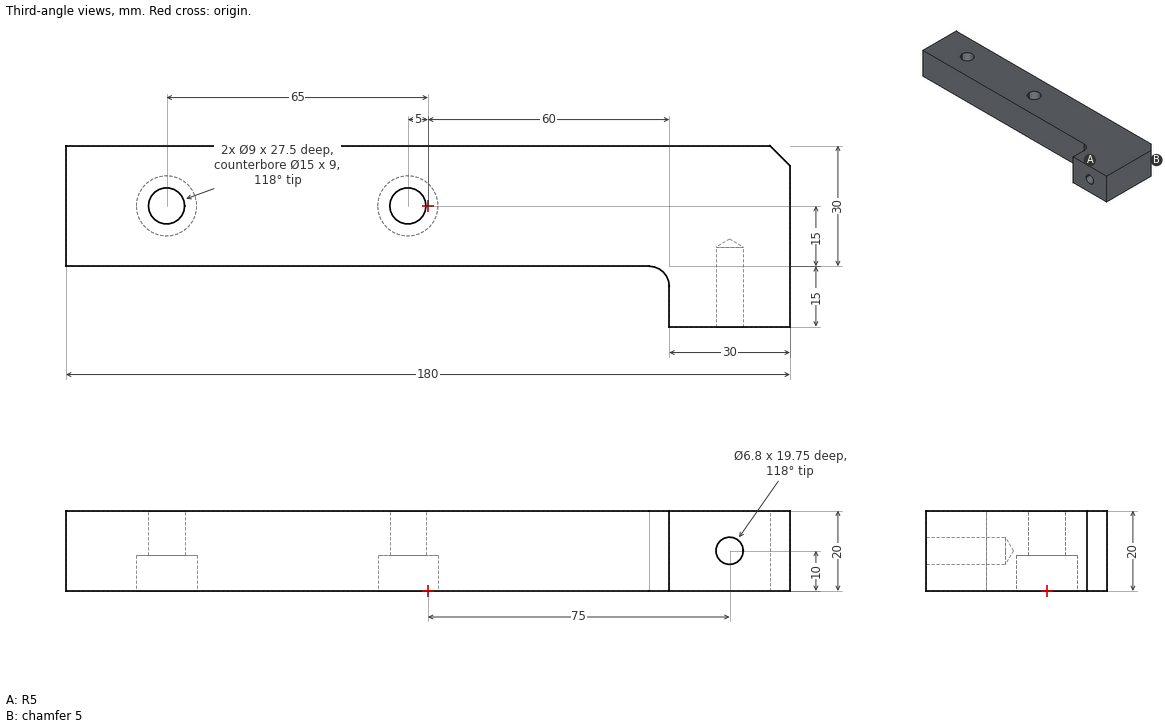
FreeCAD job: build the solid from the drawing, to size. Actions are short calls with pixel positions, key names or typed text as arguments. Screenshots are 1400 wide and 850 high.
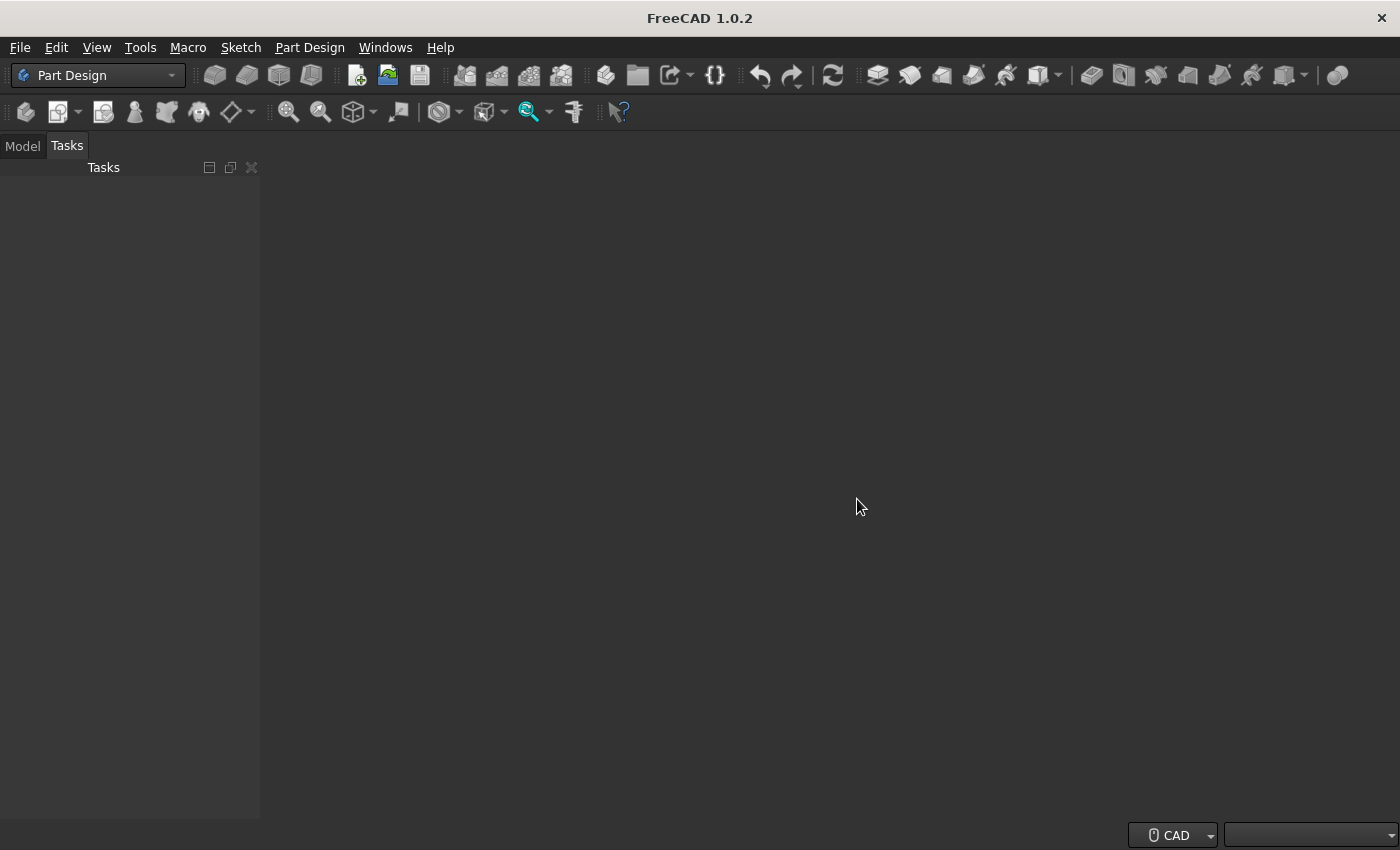
click(356, 76)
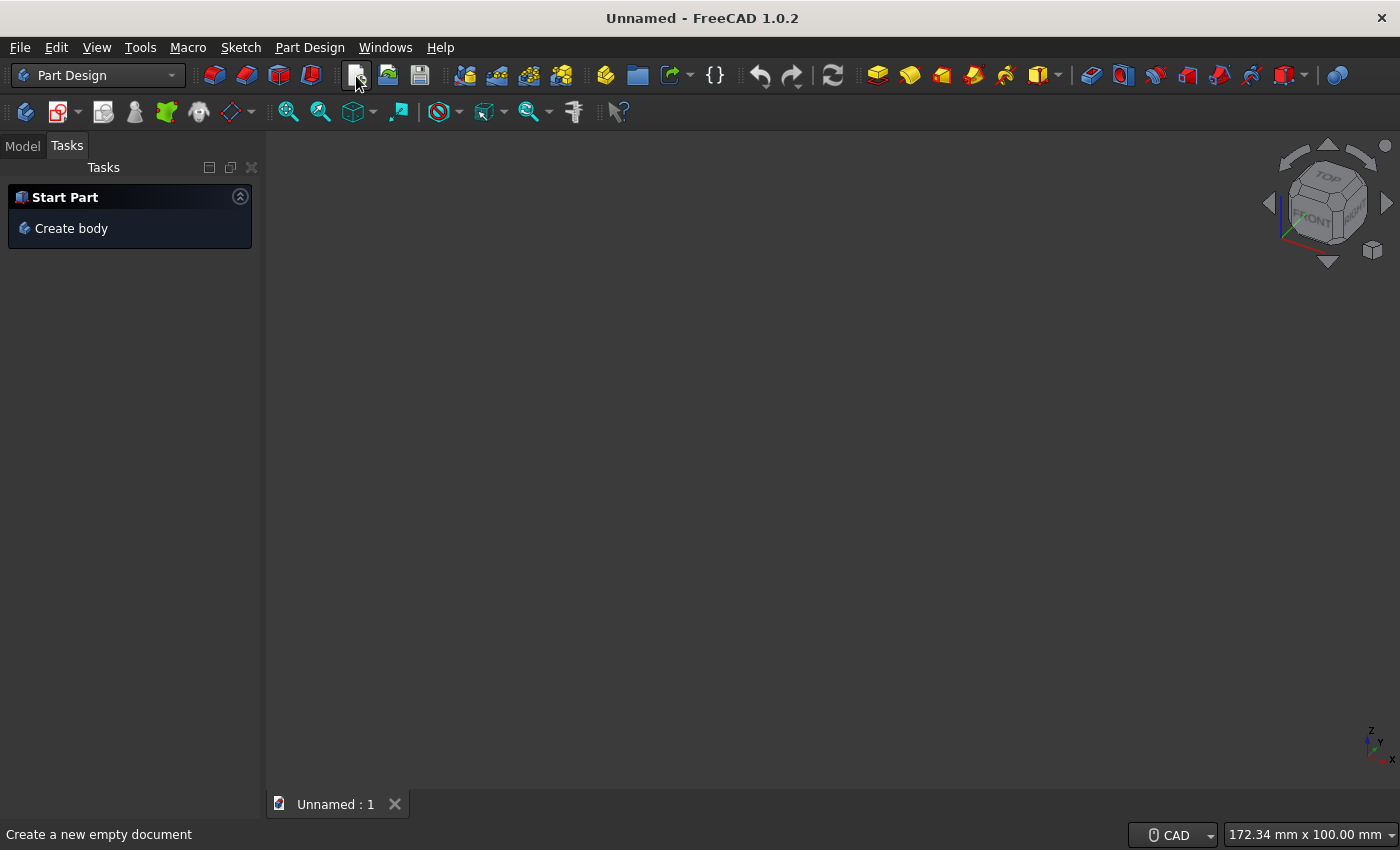
click(58, 112)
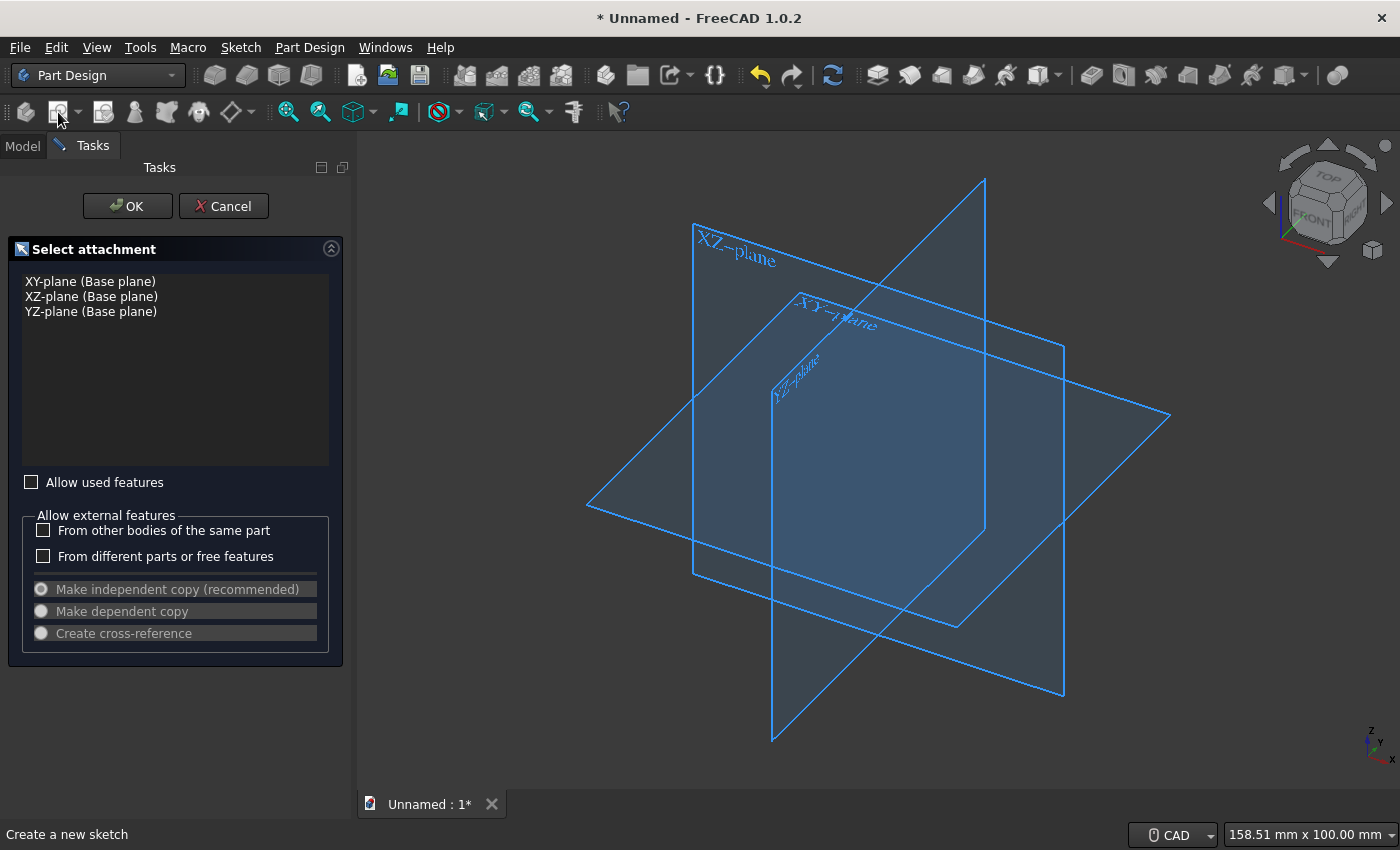
click(82, 282)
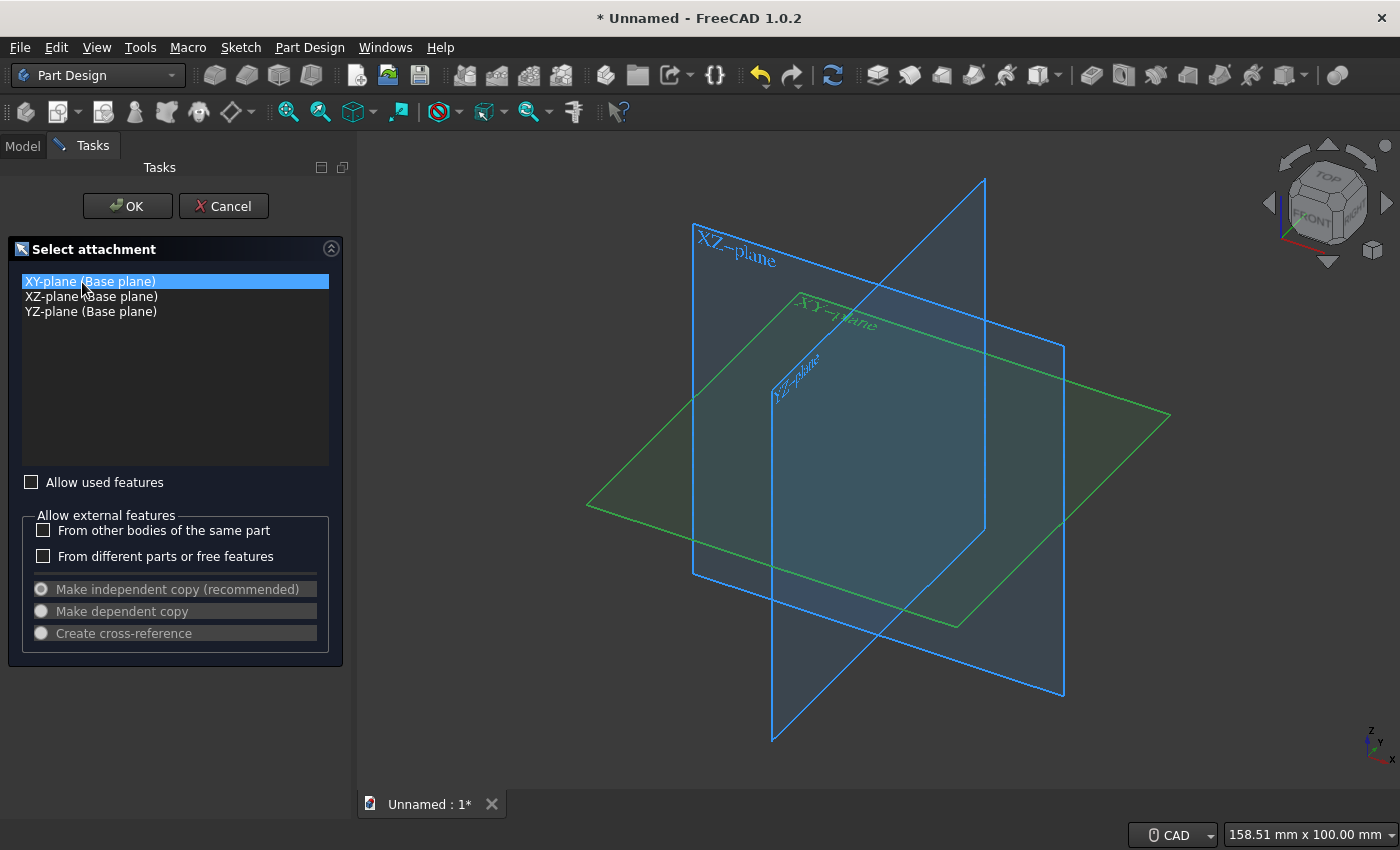
click(128, 206)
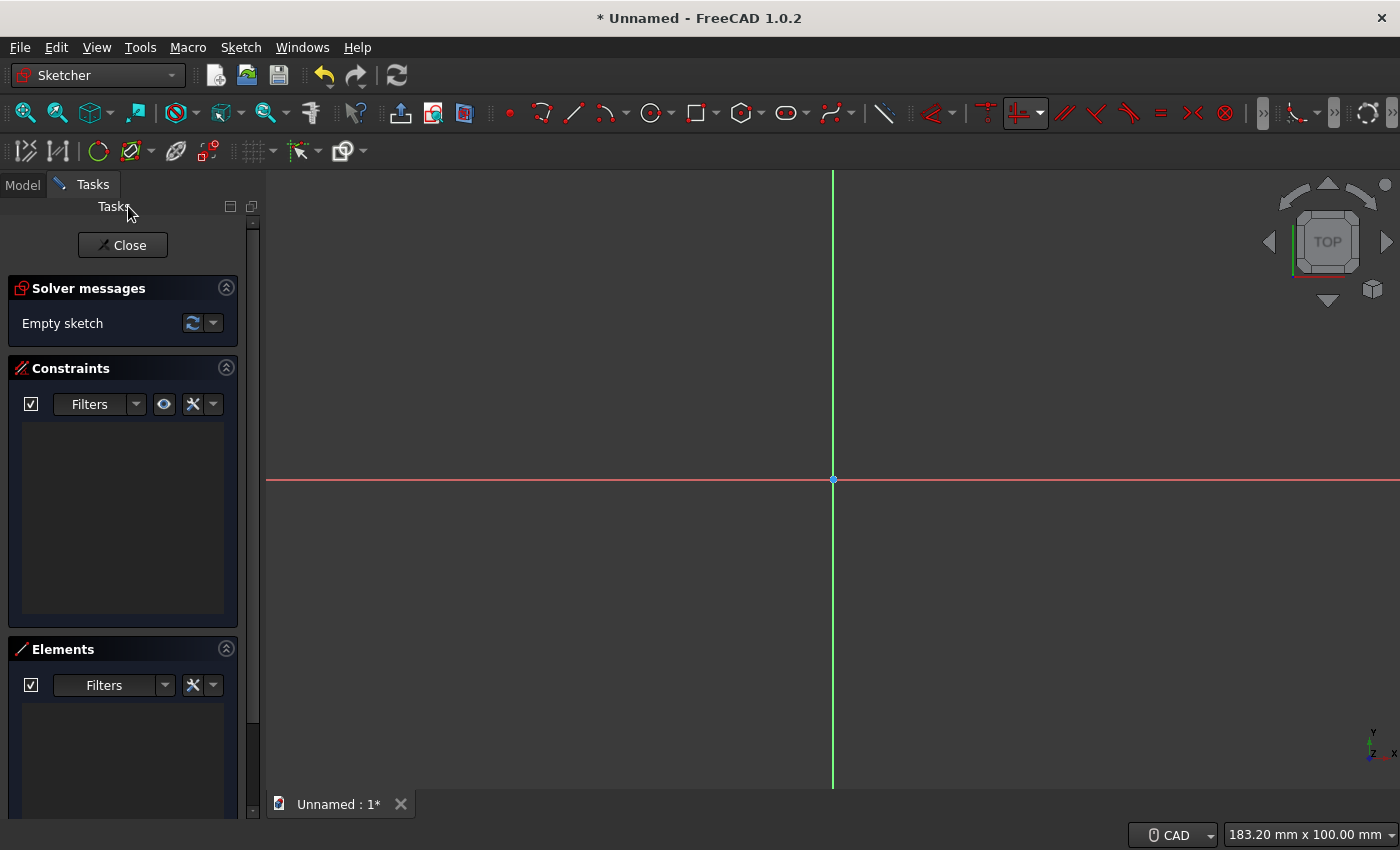
scroll(681, 479, down, 3)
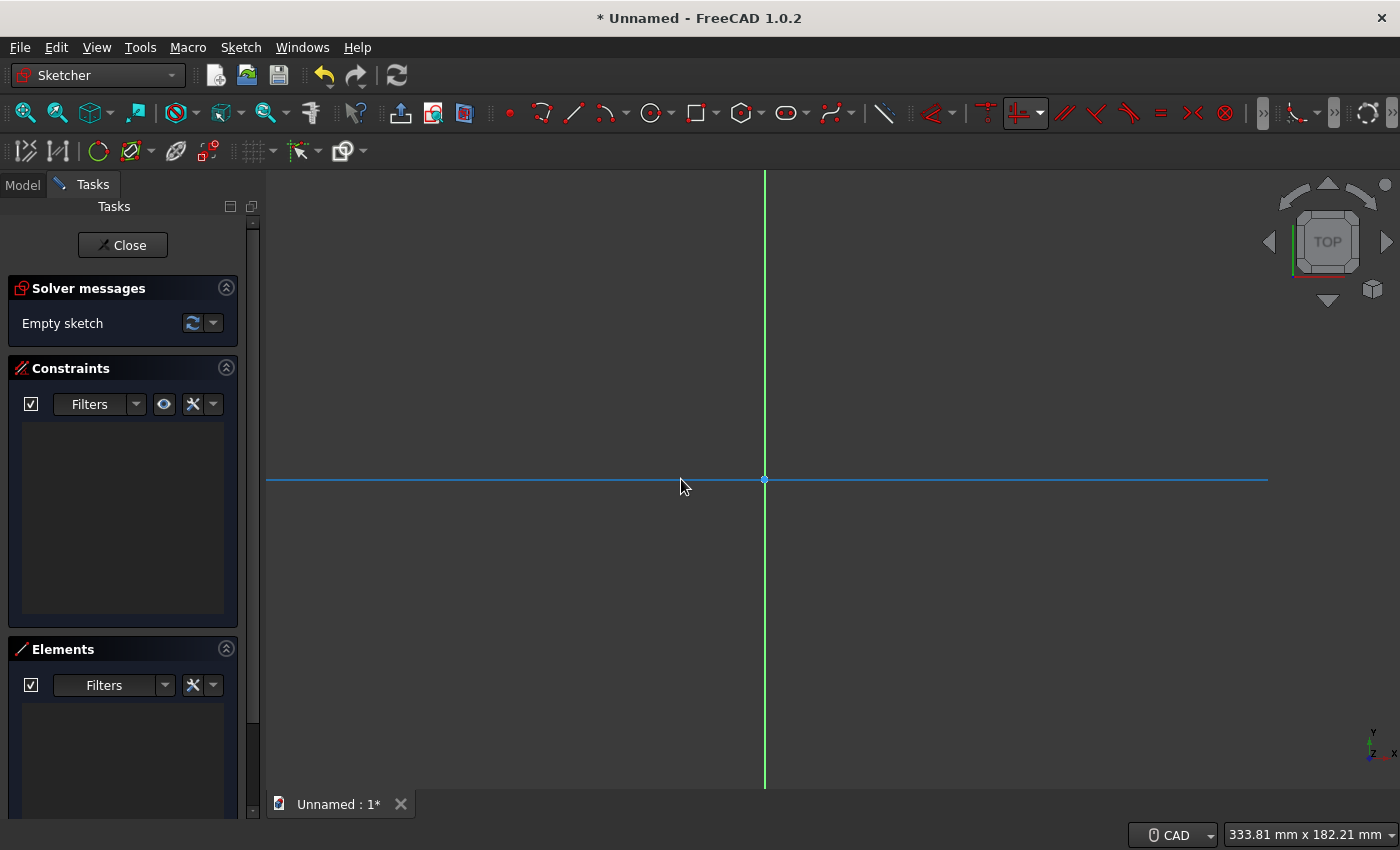
click(718, 114)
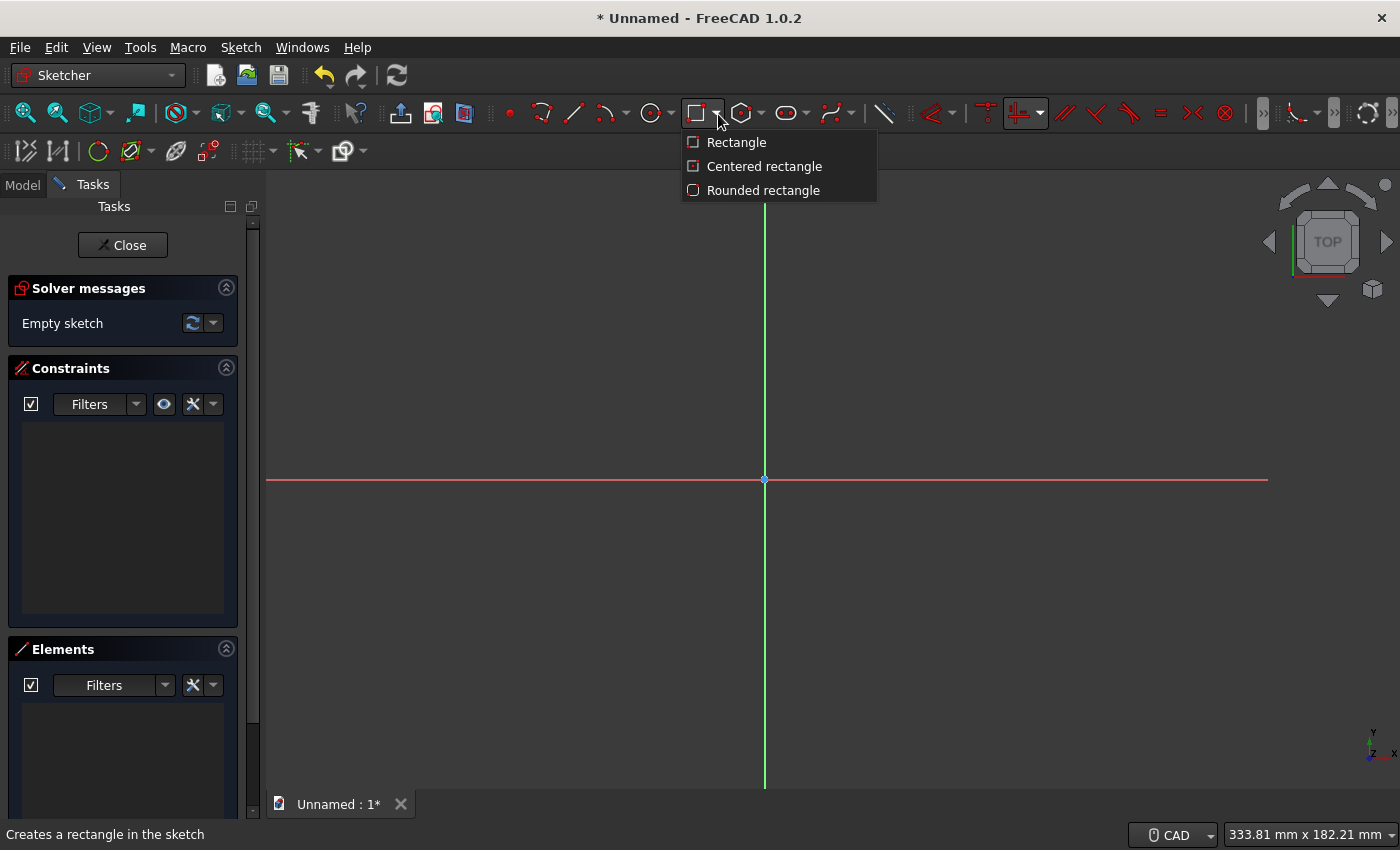
click(780, 166)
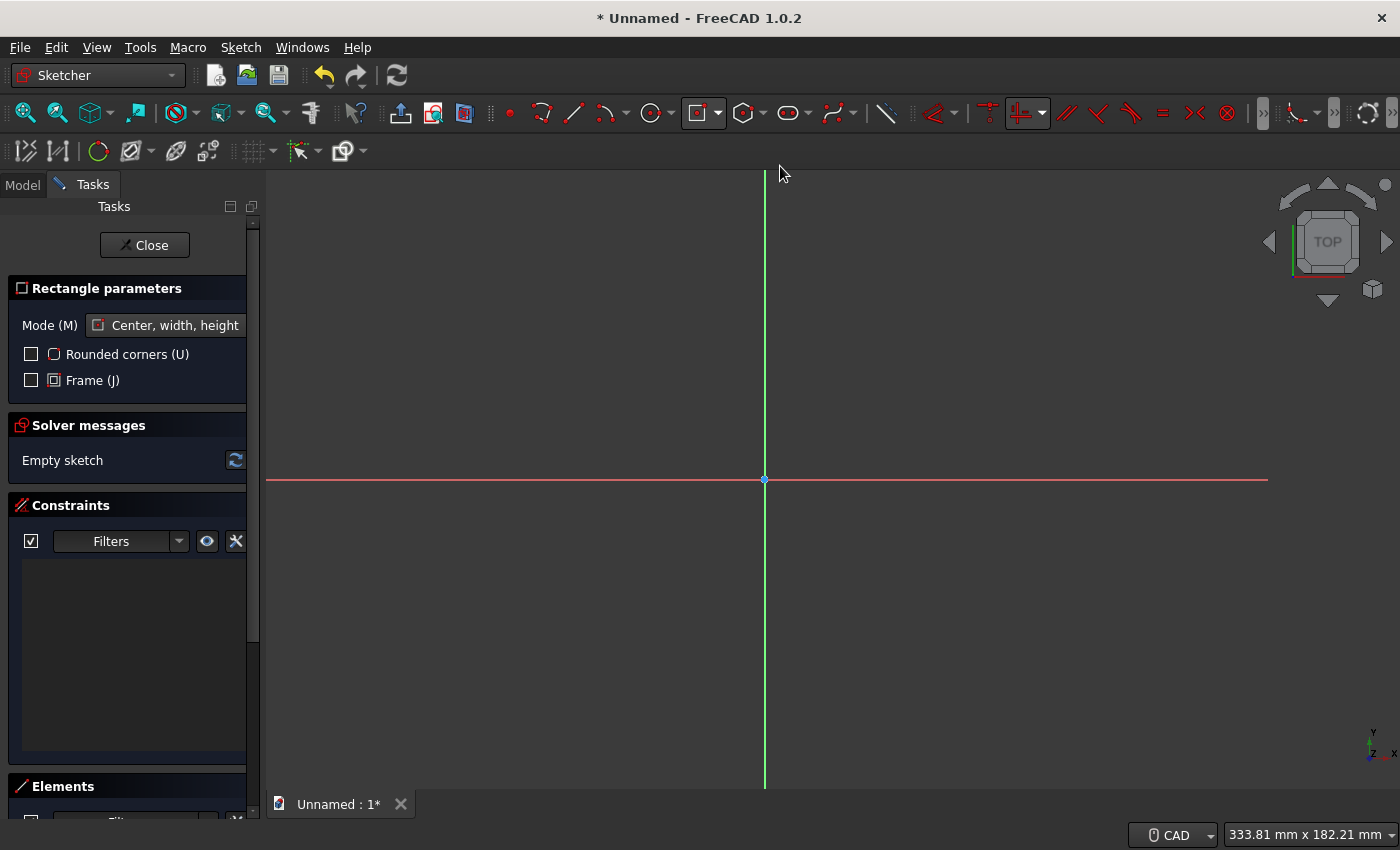
click(765, 480)
move(1070, 429)